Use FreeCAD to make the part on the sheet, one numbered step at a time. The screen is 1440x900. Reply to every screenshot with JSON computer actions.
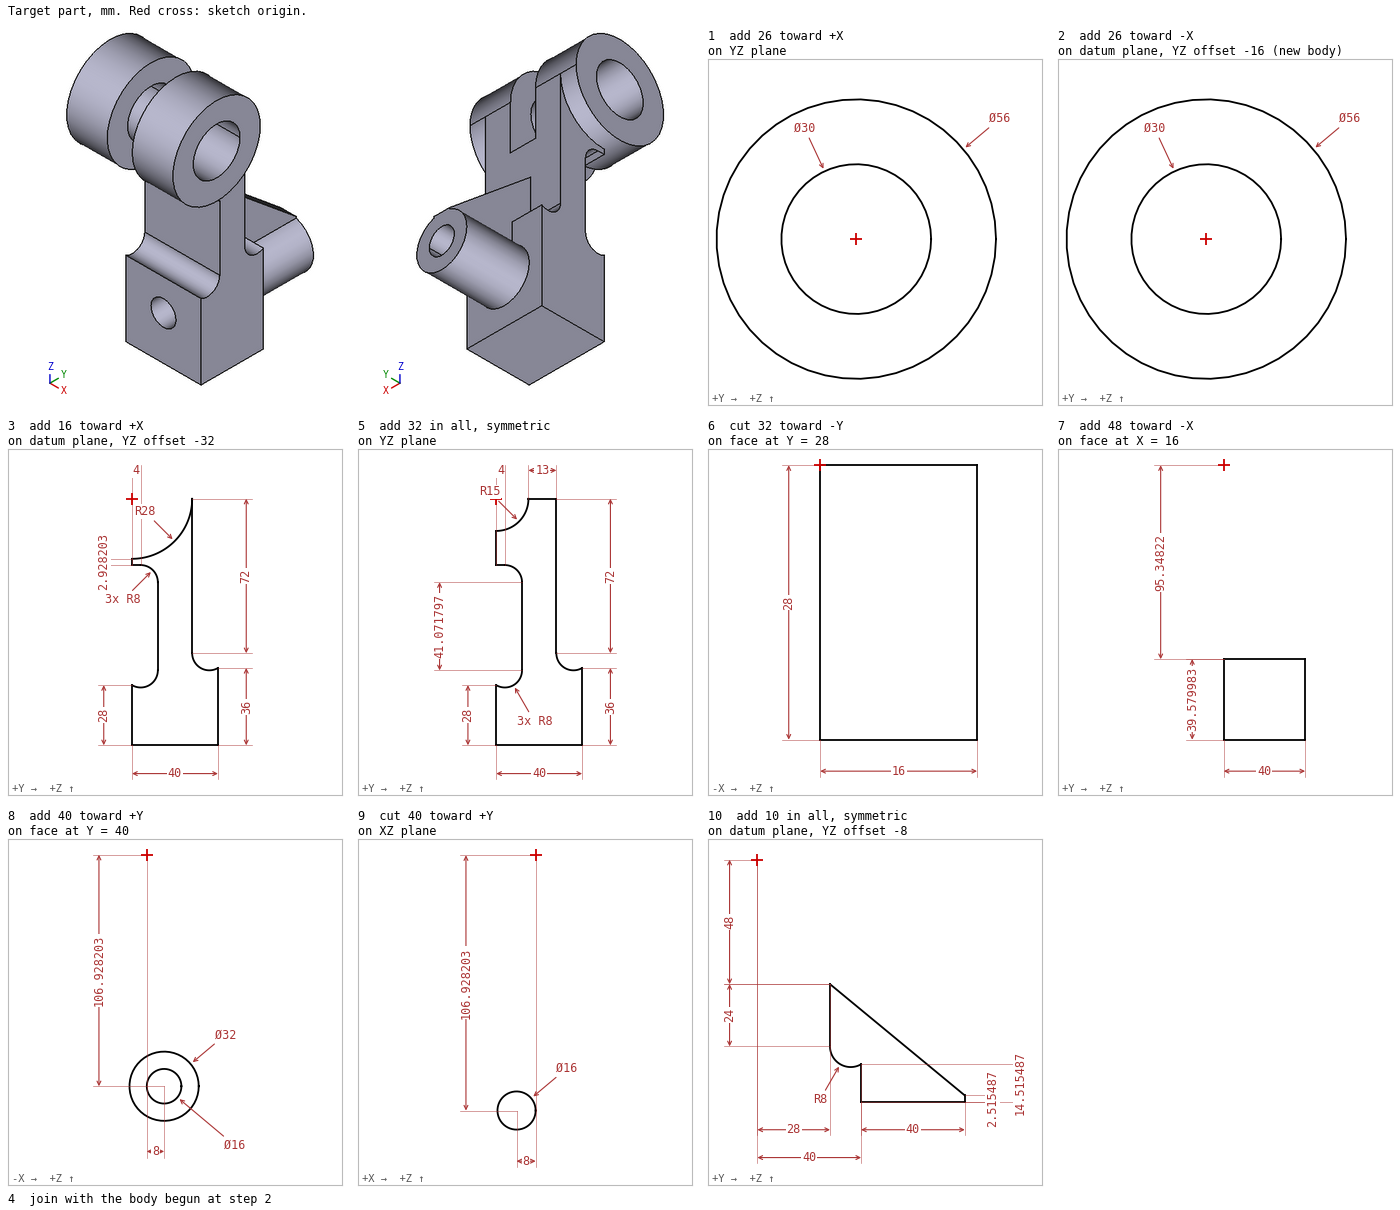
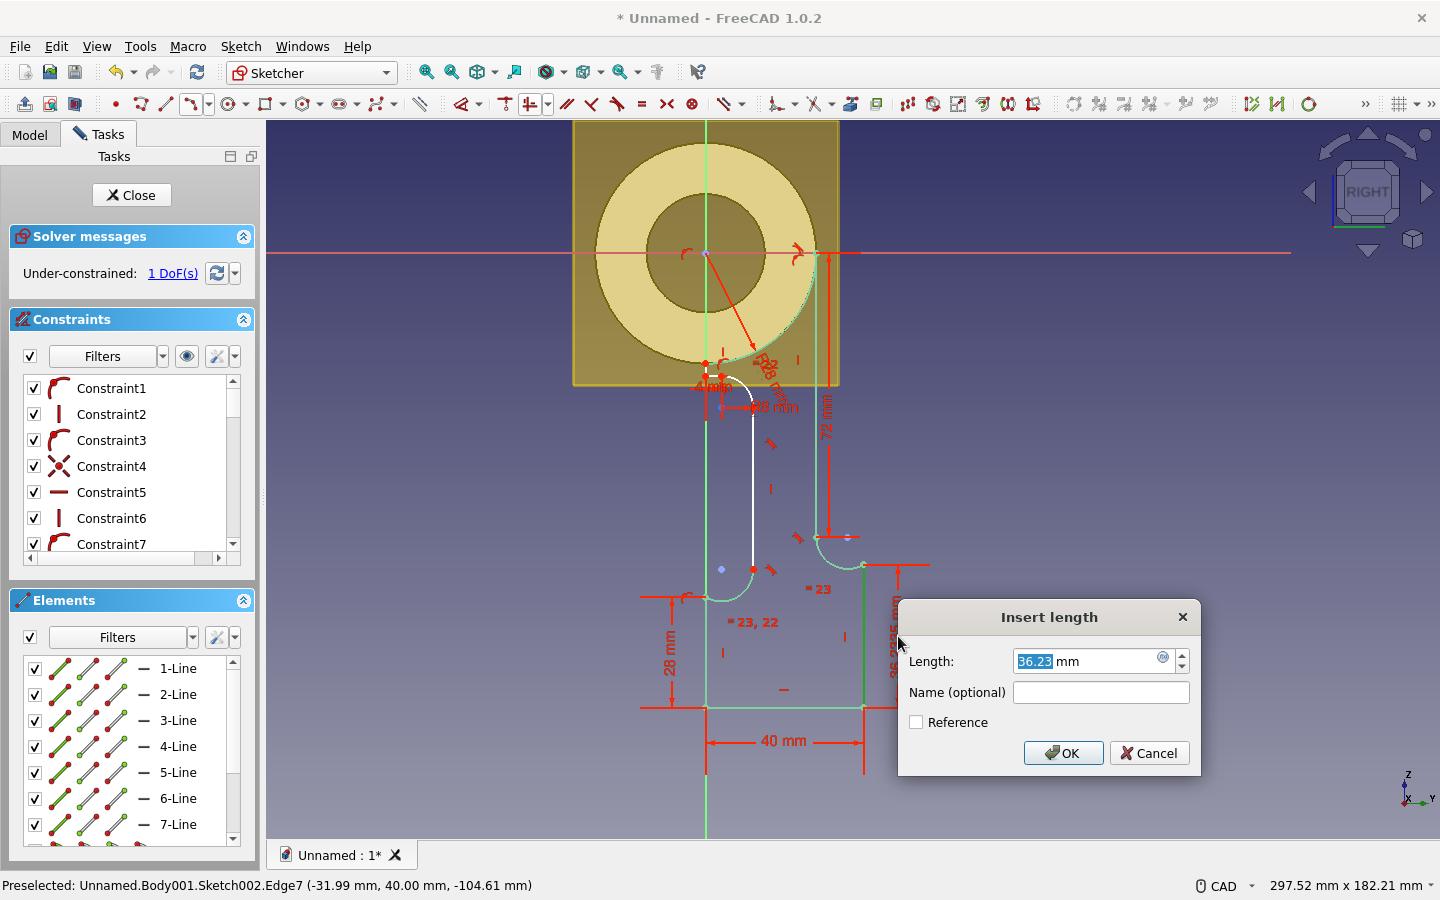
{"action": "type", "text": "36"}
{"action": "key", "text": "Return"}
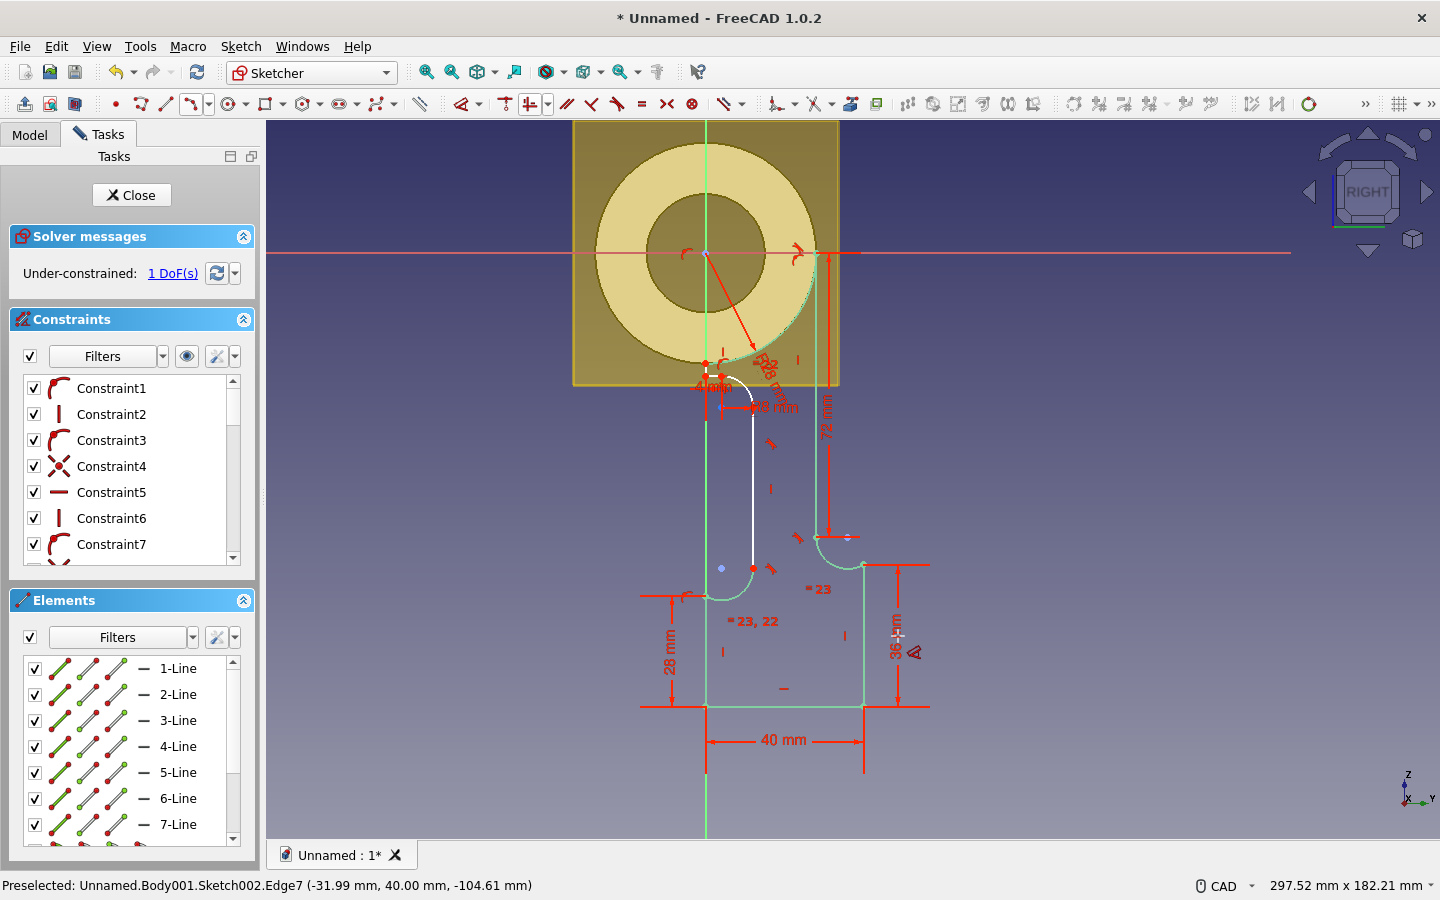
{"action": "scroll", "coordinate": [706, 370], "scroll_direction": "up", "scroll_amount": 7}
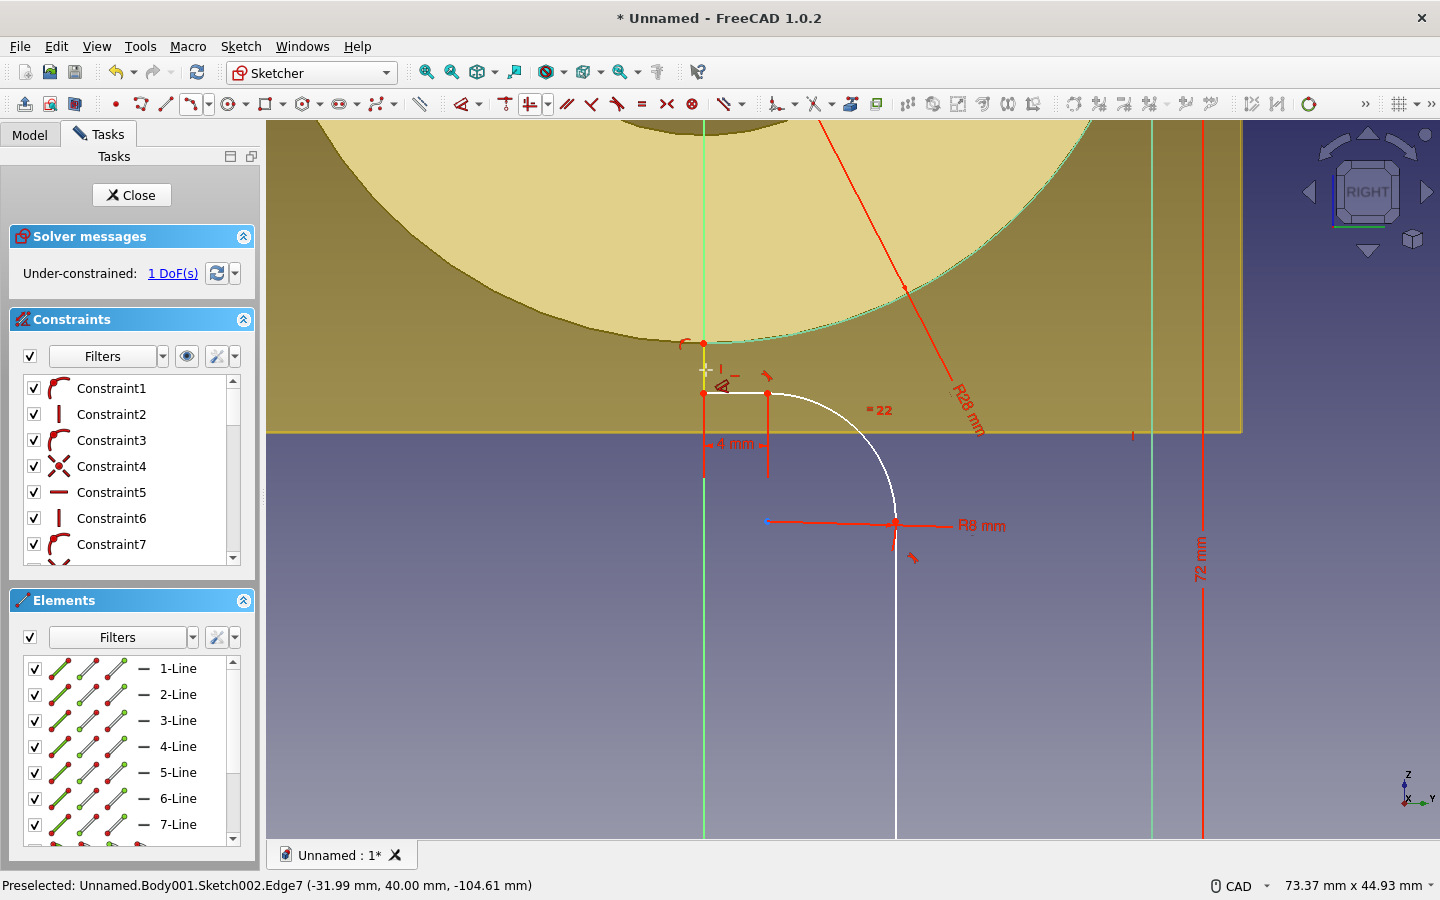
{"action": "left_click", "coordinate": [704, 368]}
{"action": "left_click", "coordinate": [670, 368]}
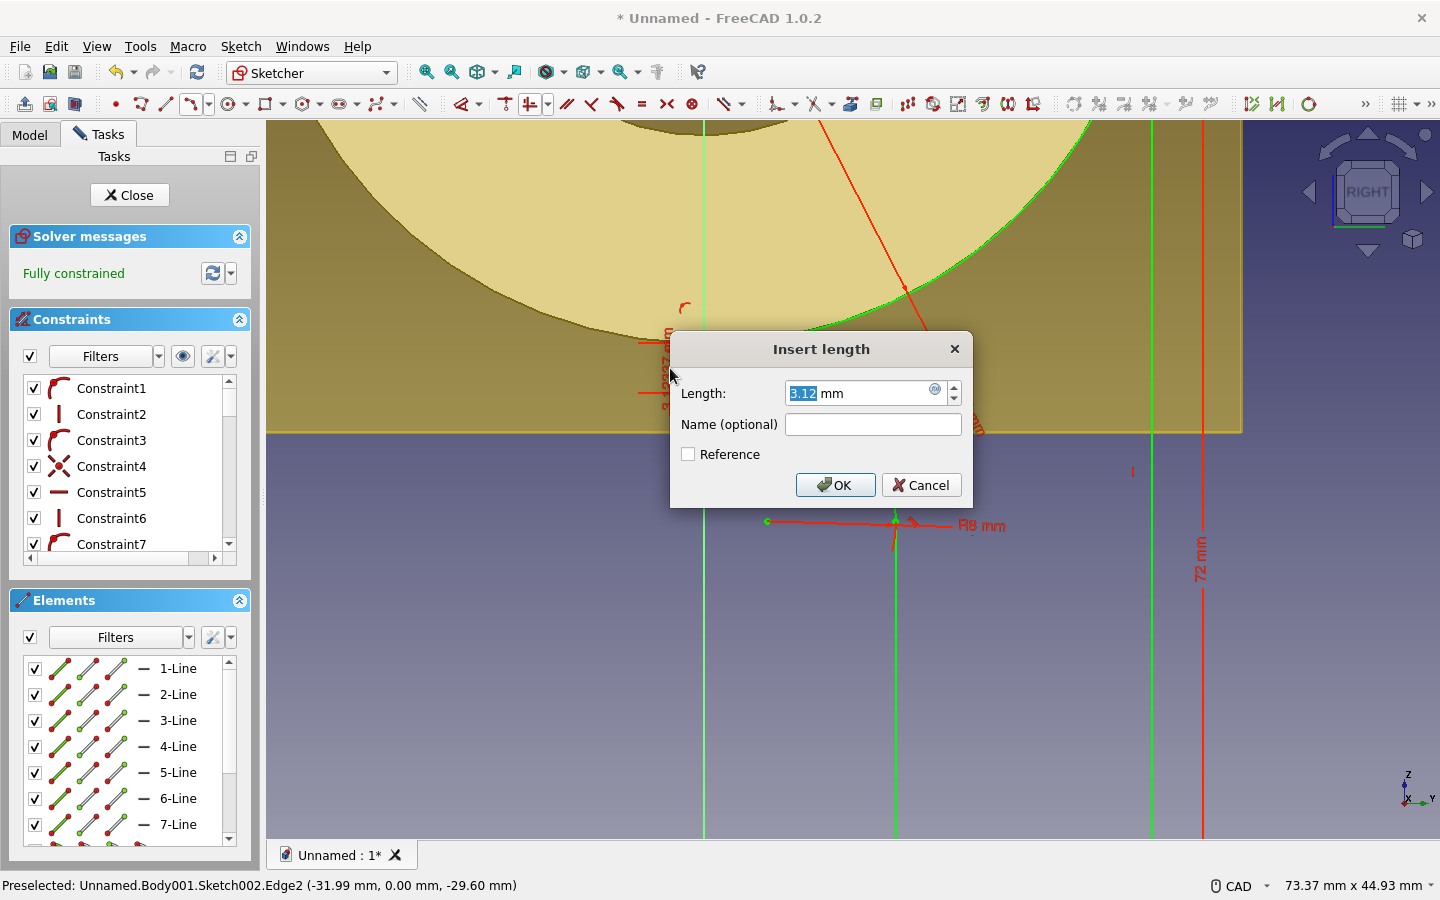
{"action": "type", "text": "2.928203"}
{"action": "key", "text": "Return"}
{"action": "key", "text": "Escape"}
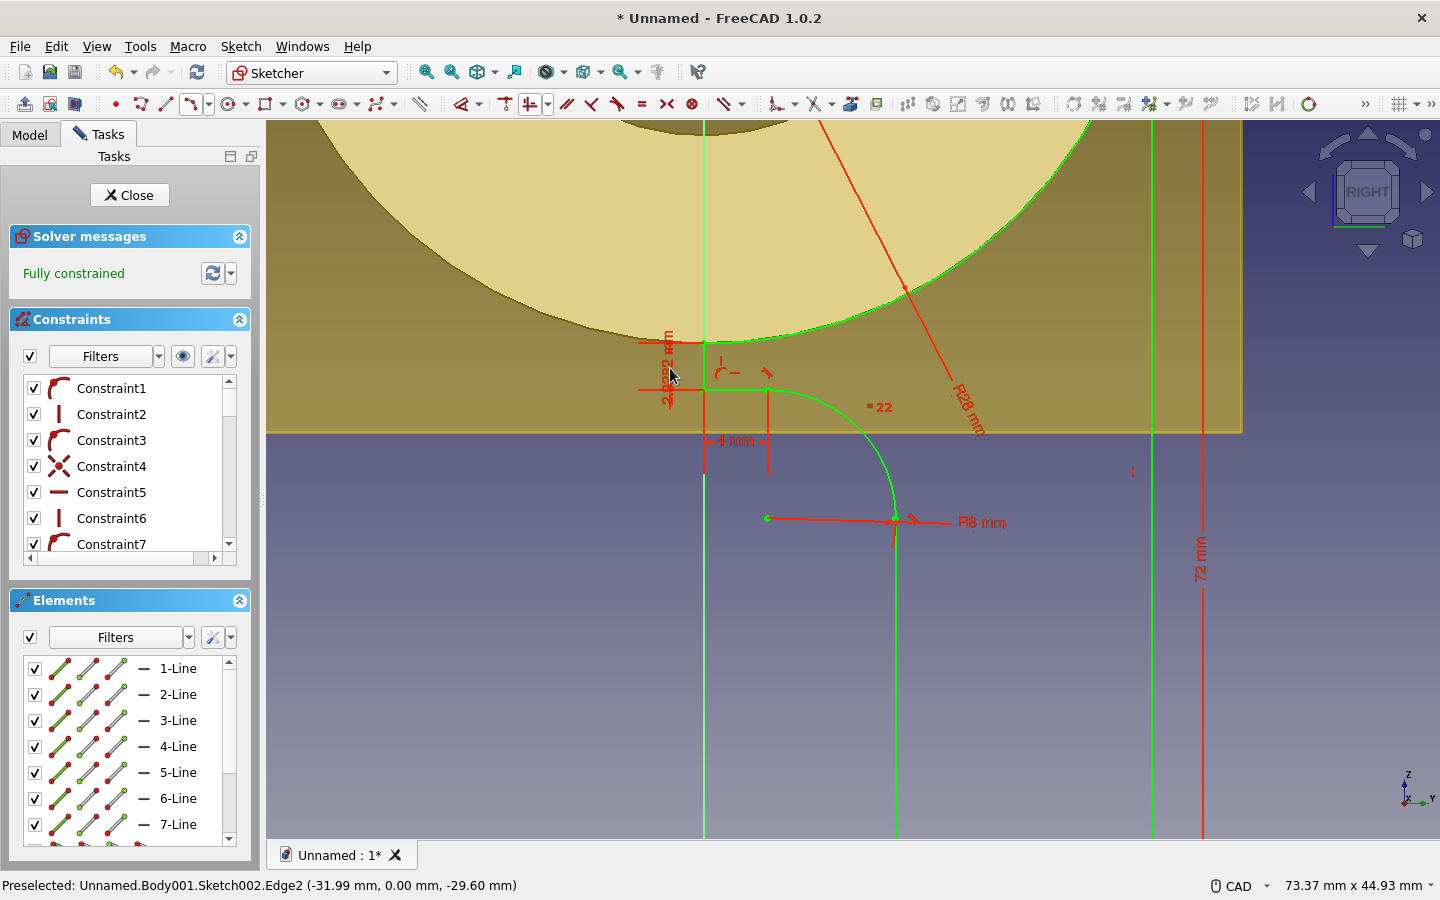
{"action": "left_click", "coordinate": [130, 195]}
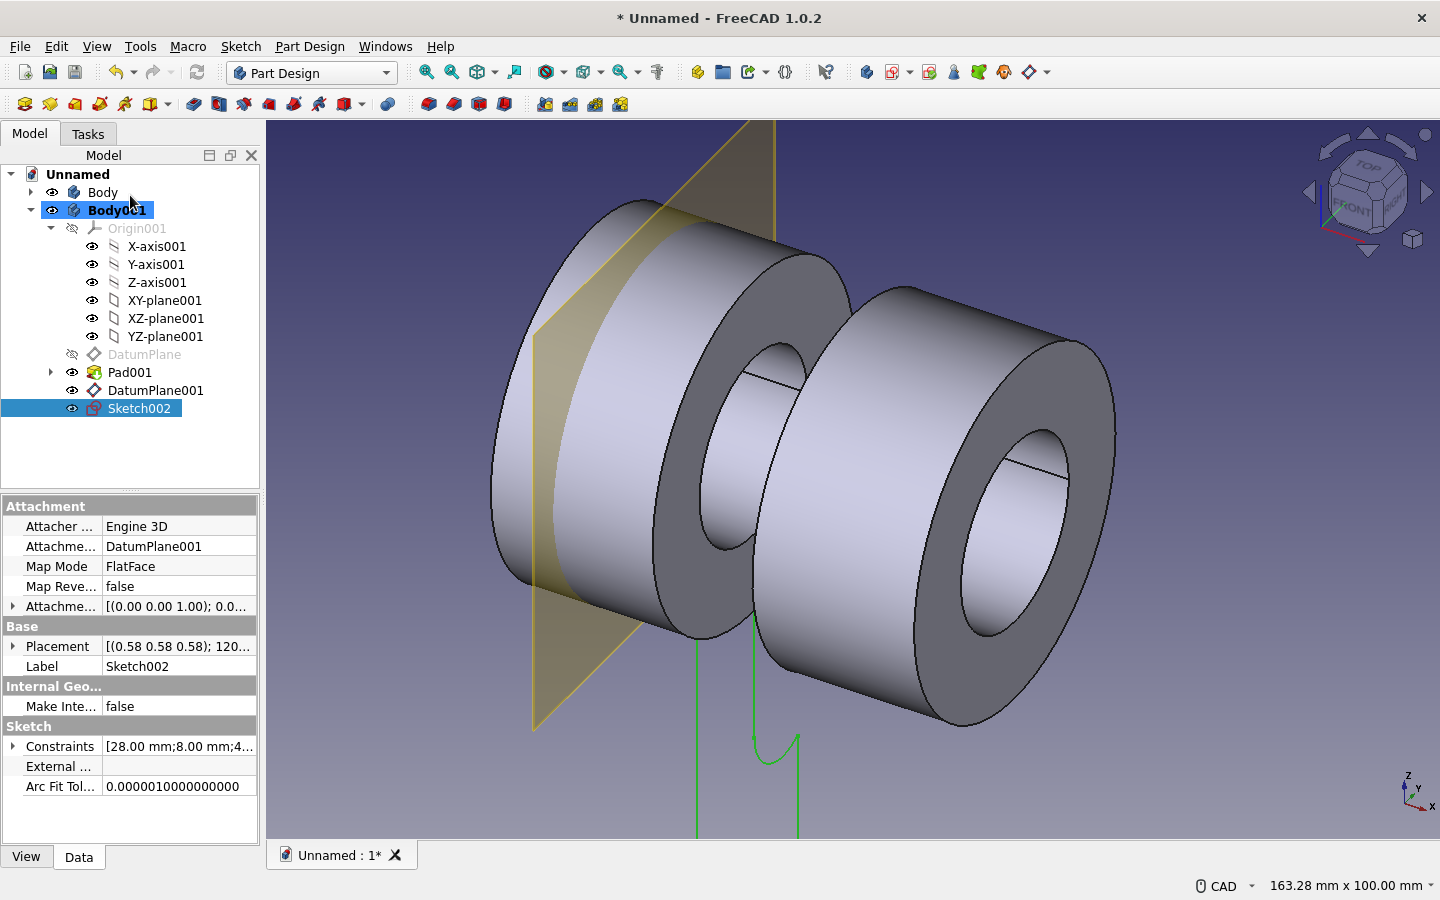
{"action": "left_click", "coordinate": [25, 104]}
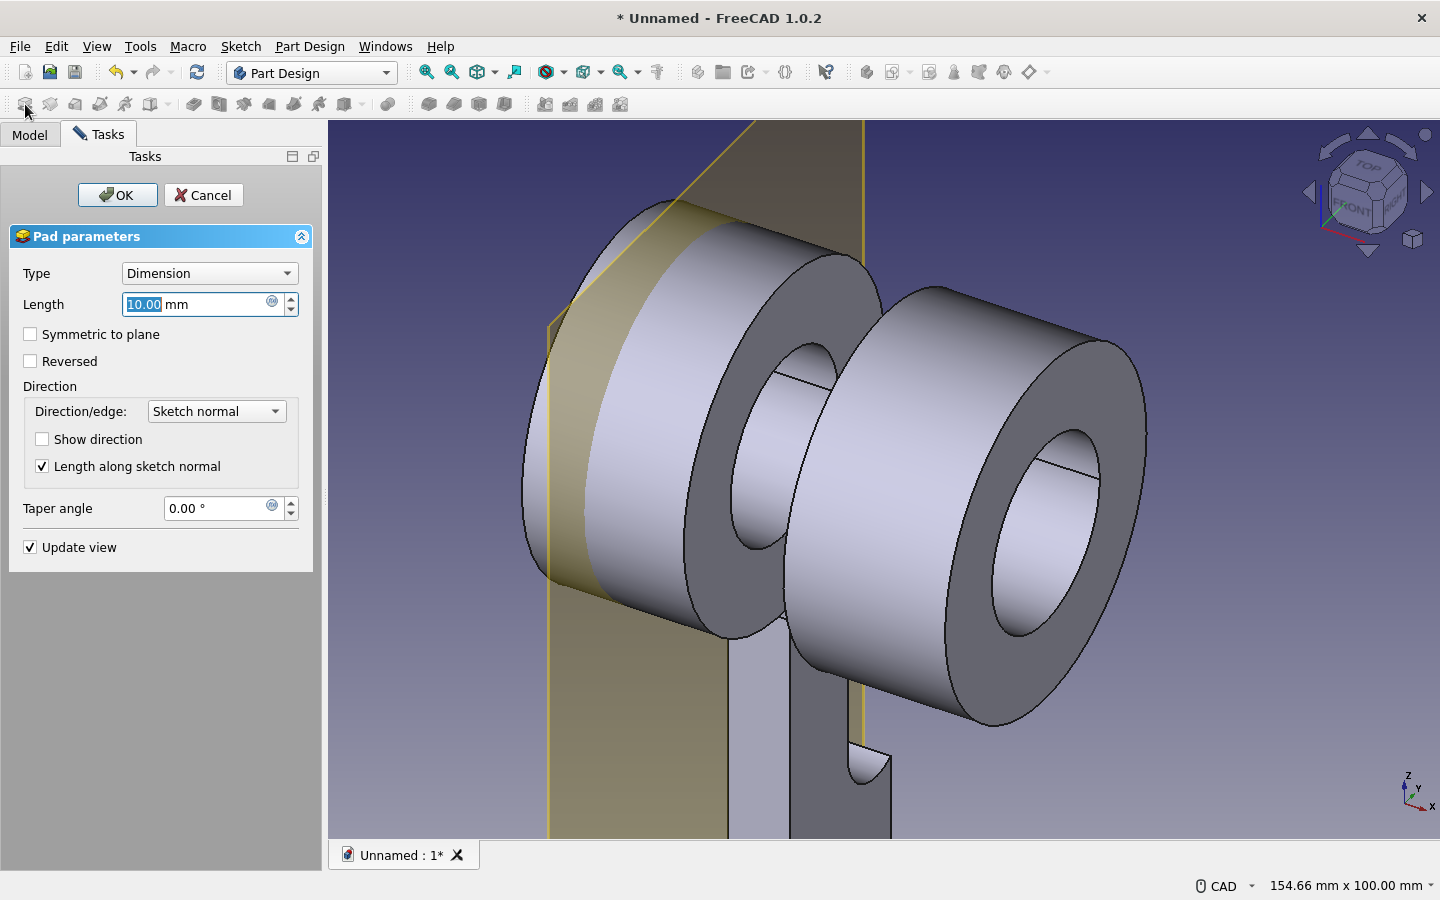
{"action": "type", "text": "16"}
{"action": "key", "text": "Tab"}